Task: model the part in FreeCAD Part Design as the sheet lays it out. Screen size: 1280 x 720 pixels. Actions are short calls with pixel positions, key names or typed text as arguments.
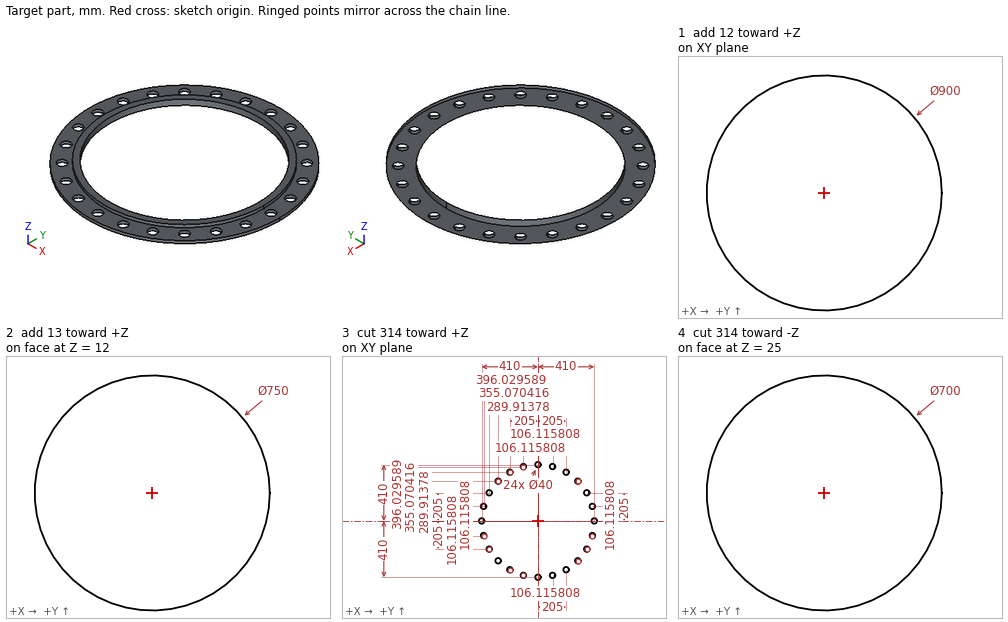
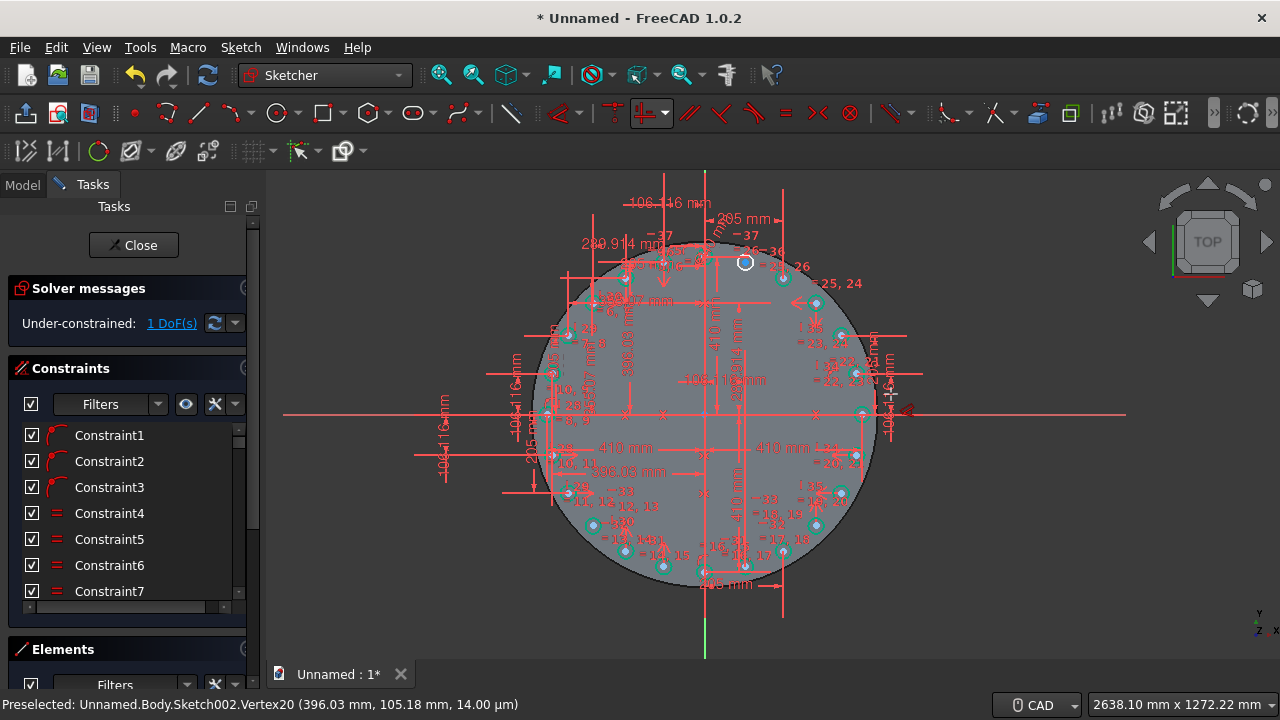
click(745, 262)
click(725, 473)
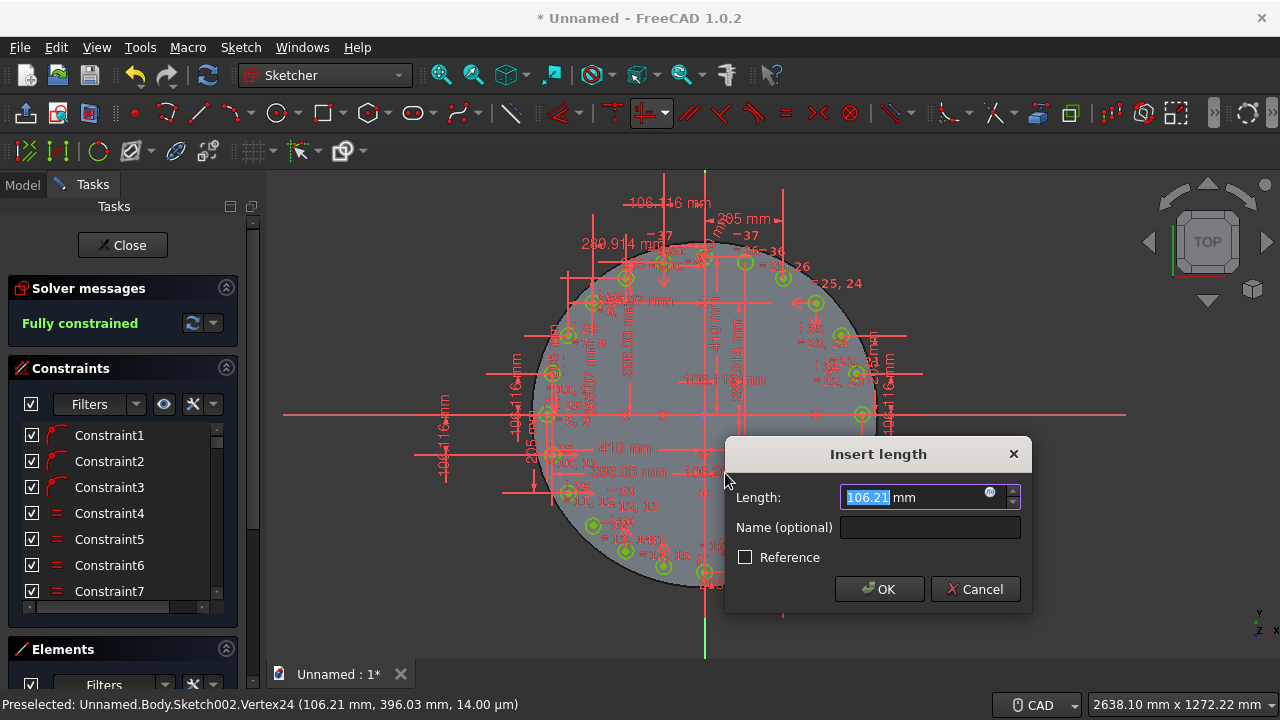
text(106.115808)
key(Return)
key(Escape)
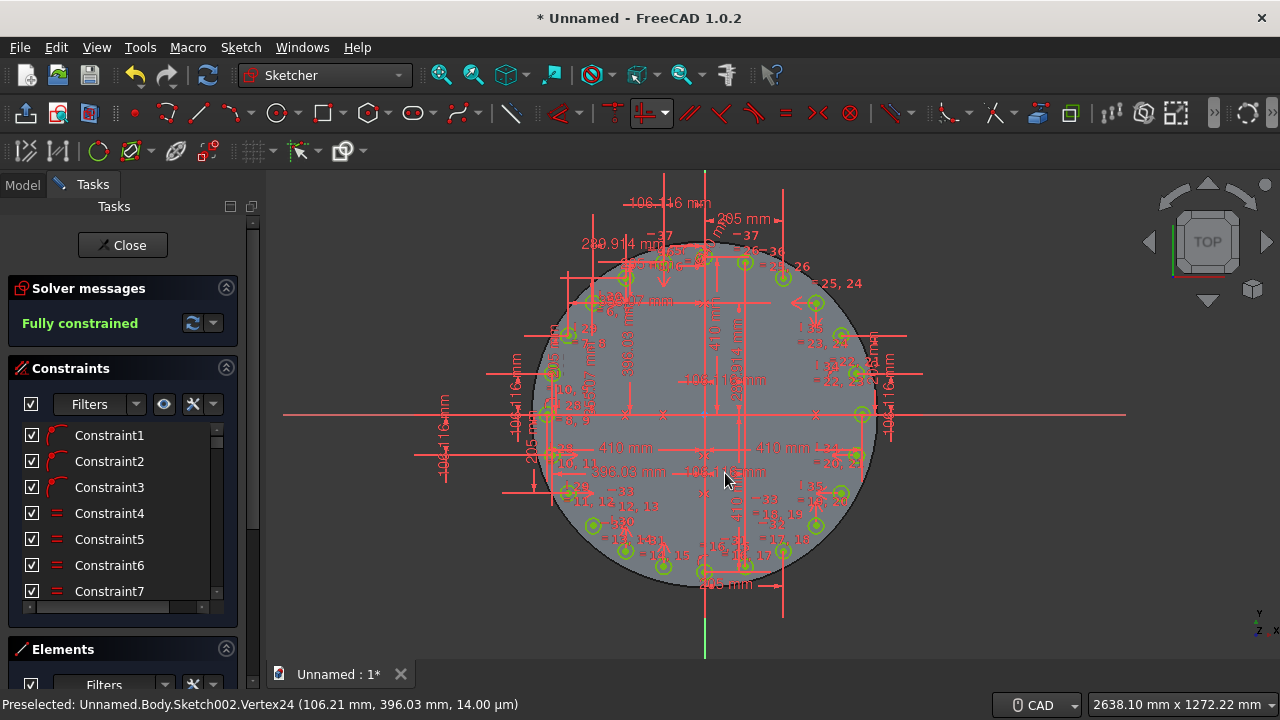
click(123, 245)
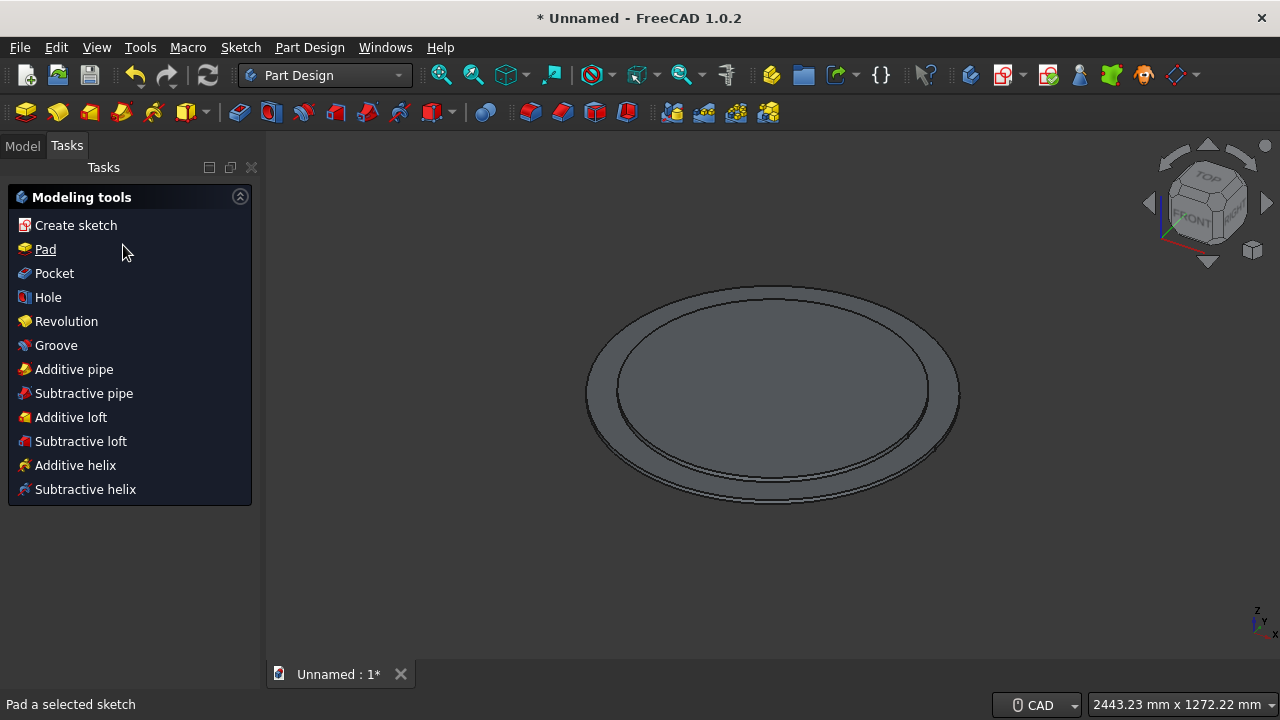
click(240, 112)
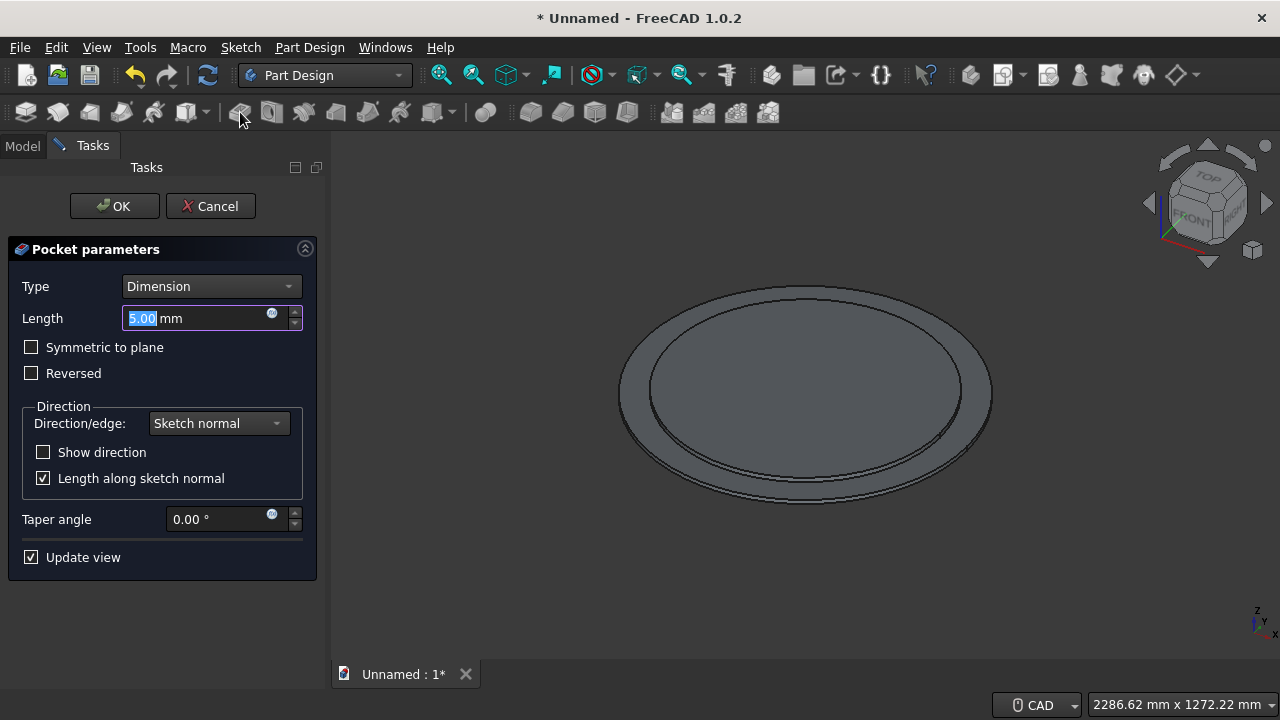
text(314)
key(Tab)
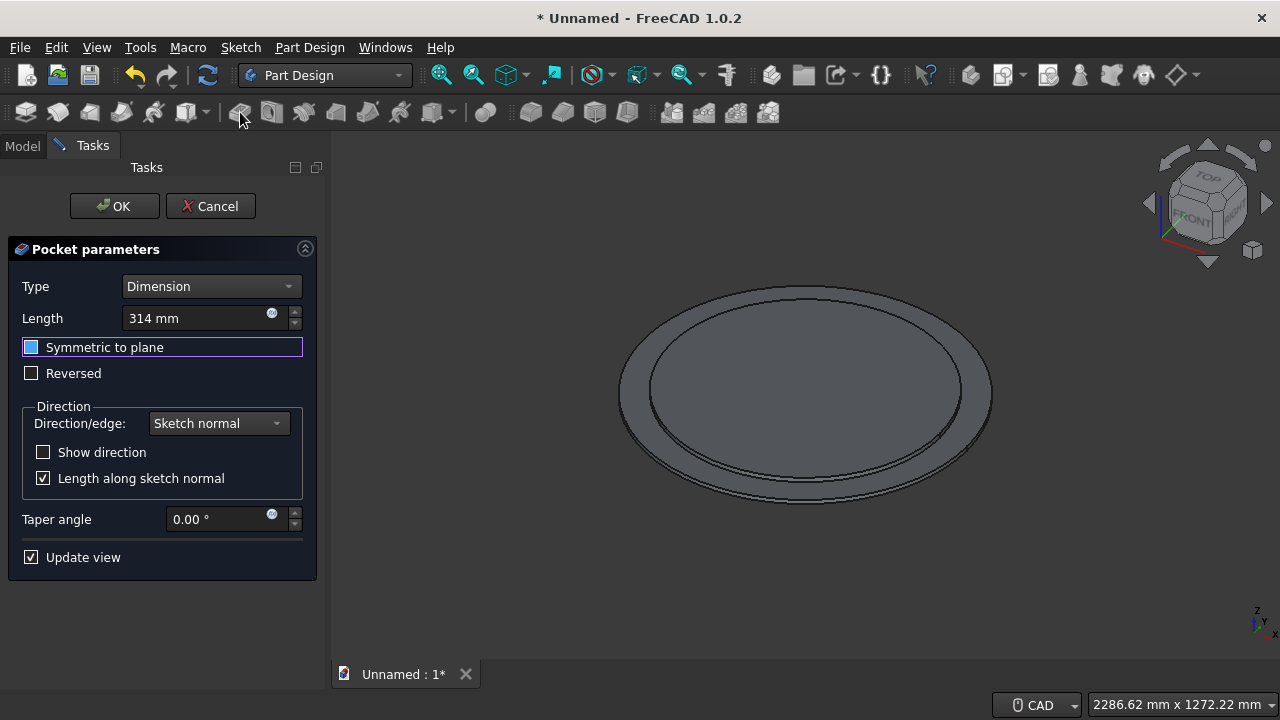
click(30, 373)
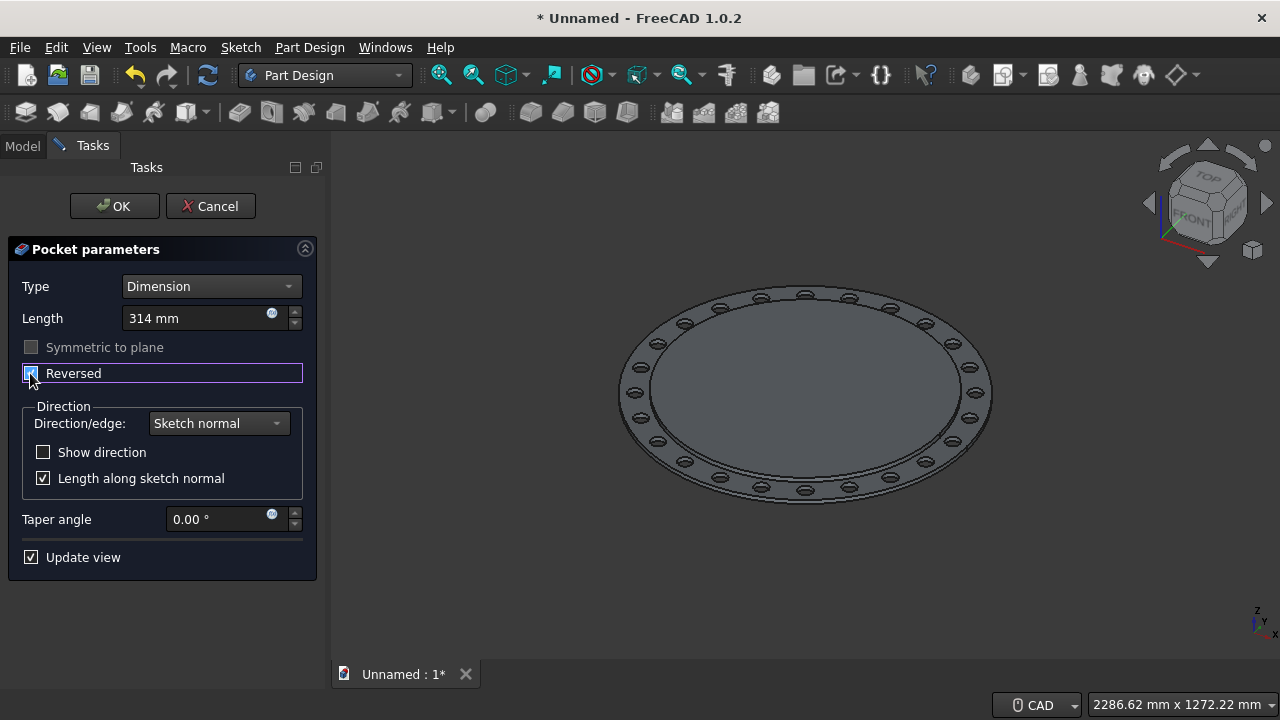
click(115, 206)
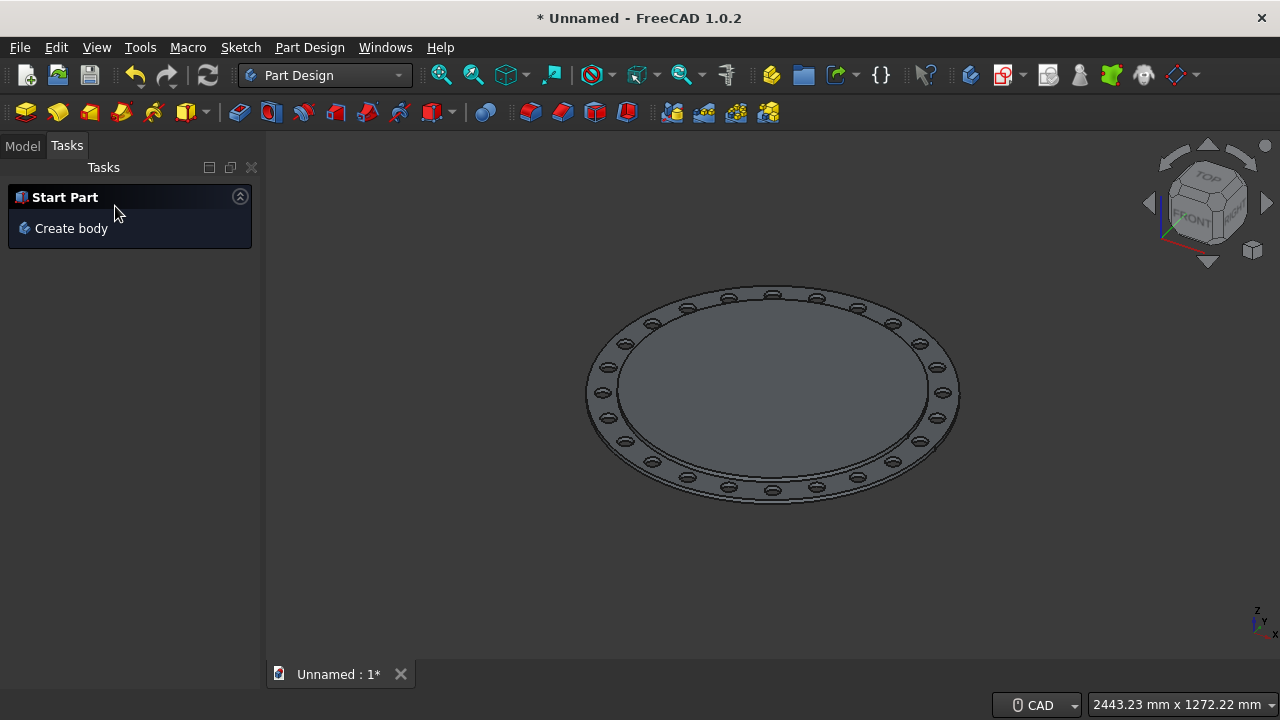
click(773, 387)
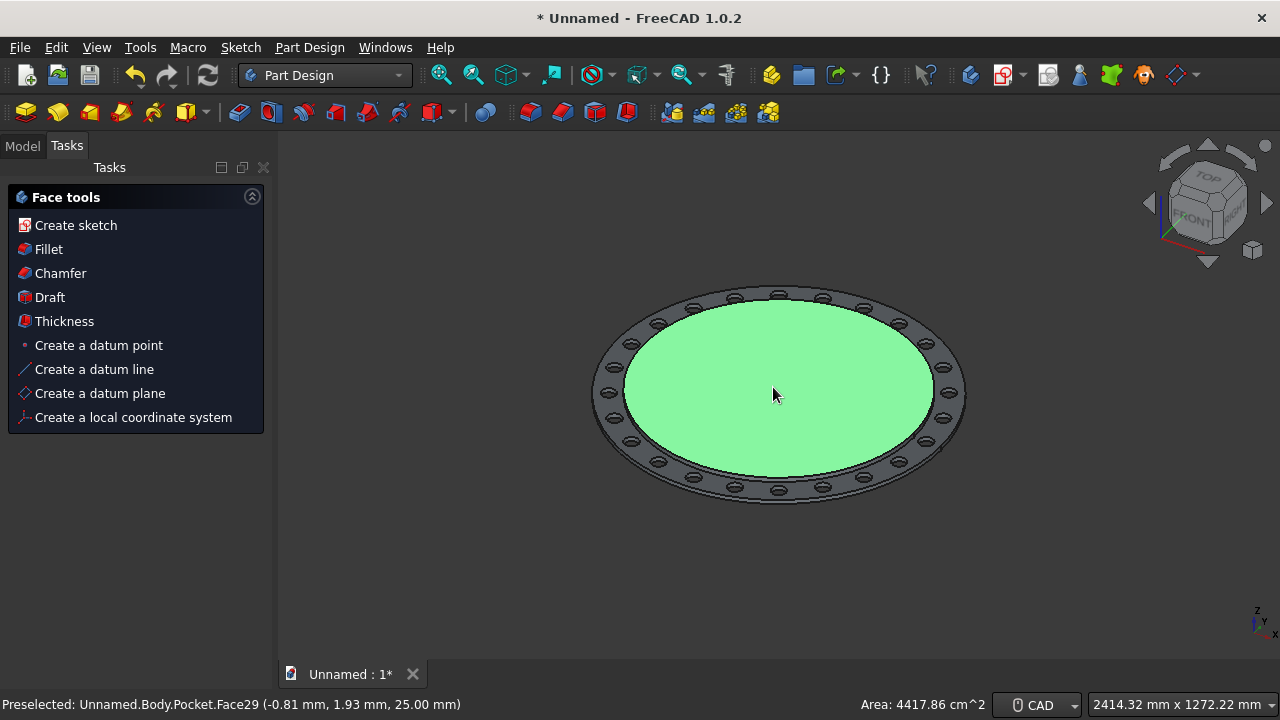
click(1004, 76)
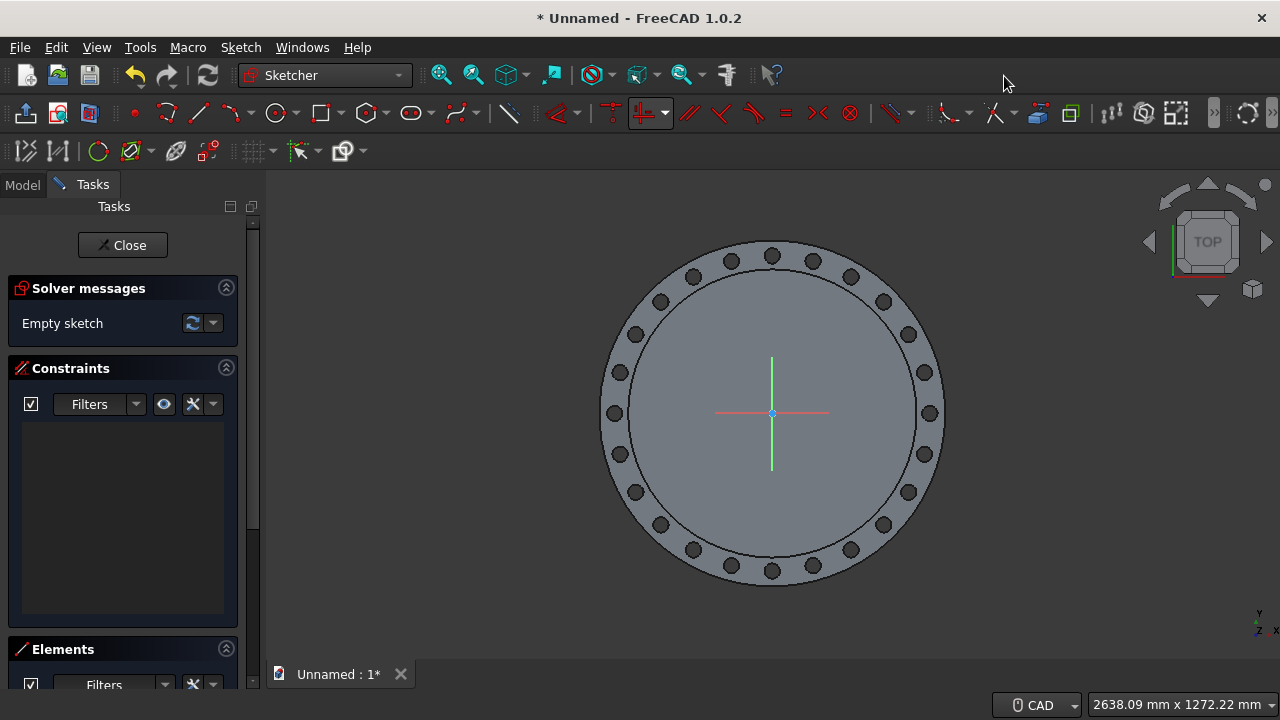
click(276, 114)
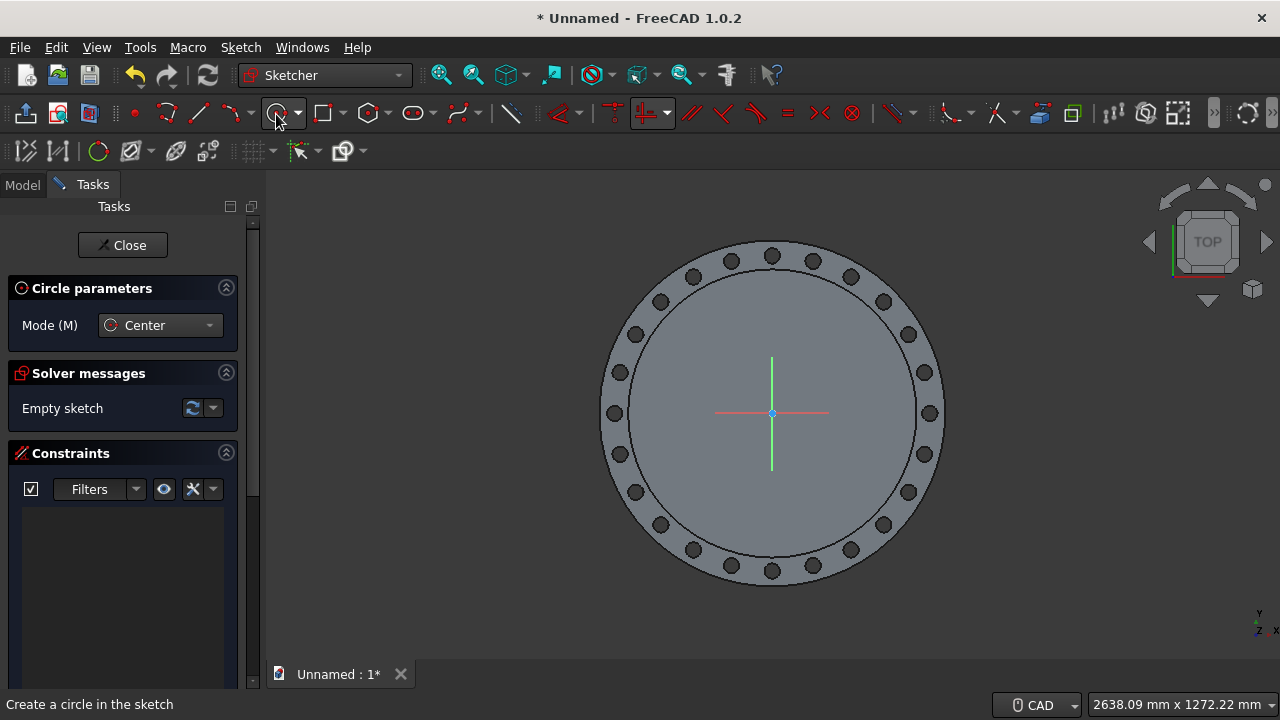
click(772, 413)
click(867, 318)
key(Escape)